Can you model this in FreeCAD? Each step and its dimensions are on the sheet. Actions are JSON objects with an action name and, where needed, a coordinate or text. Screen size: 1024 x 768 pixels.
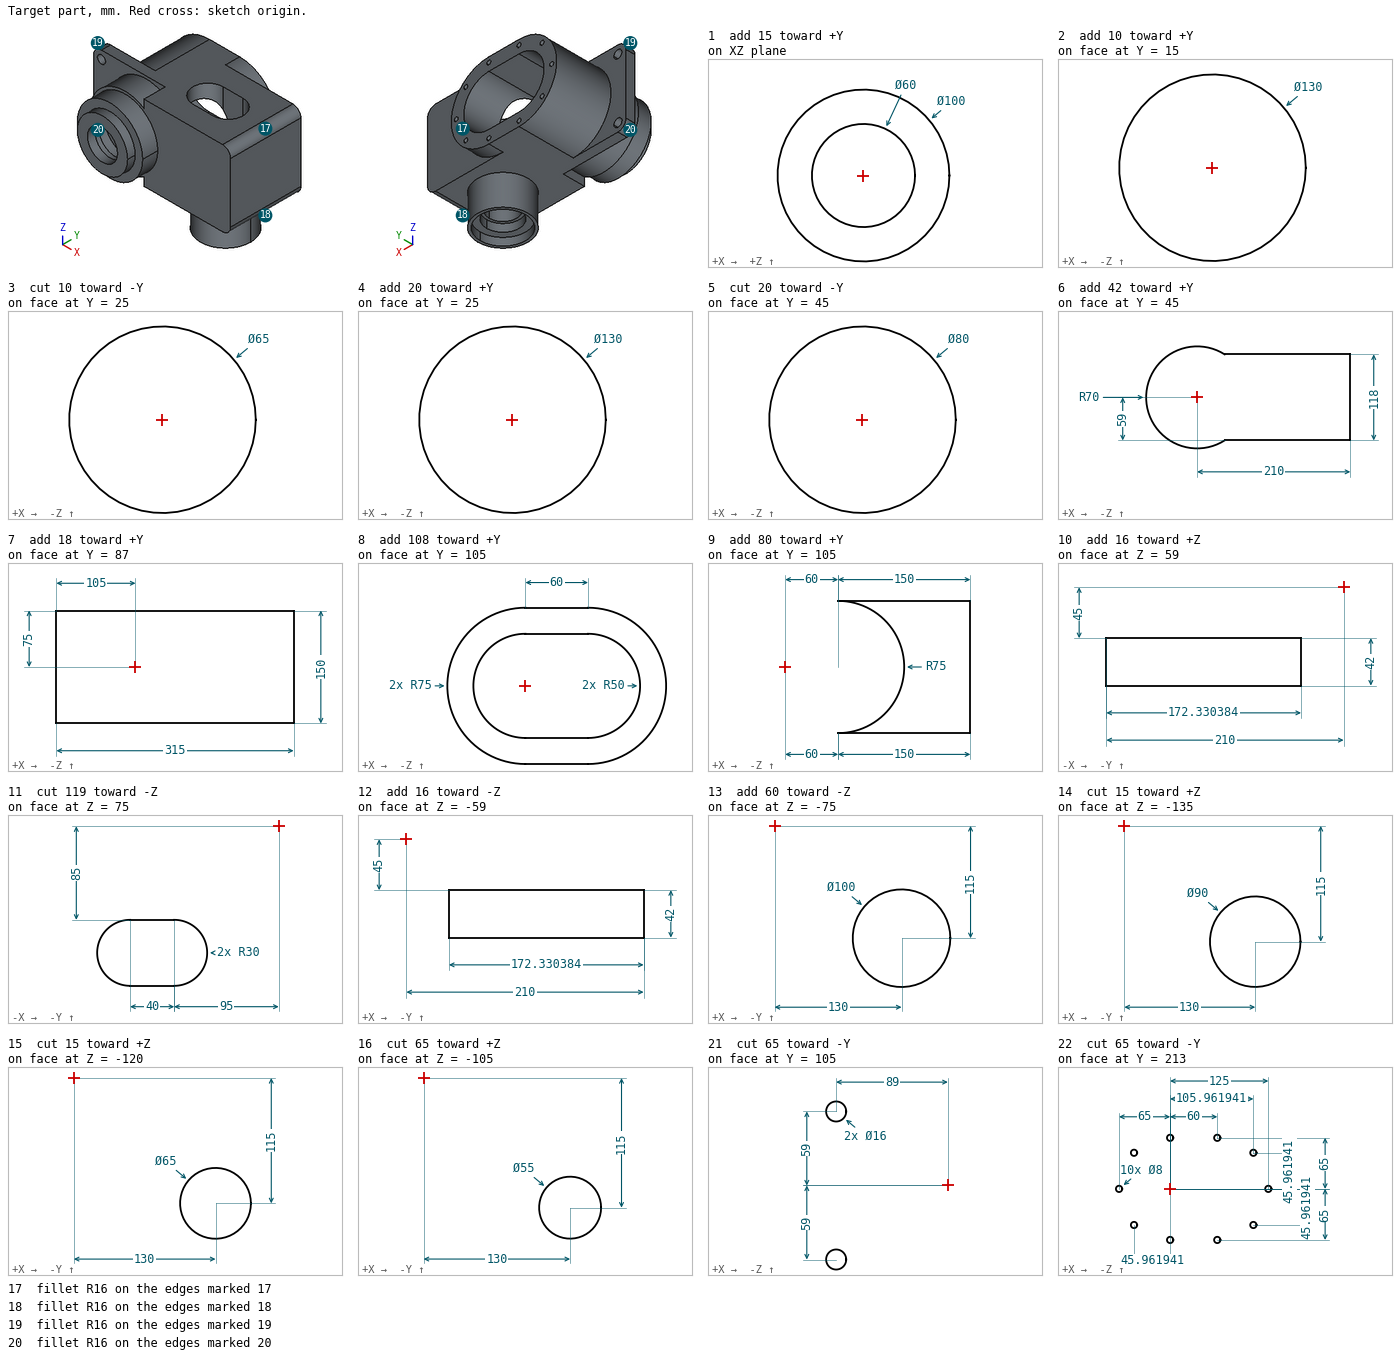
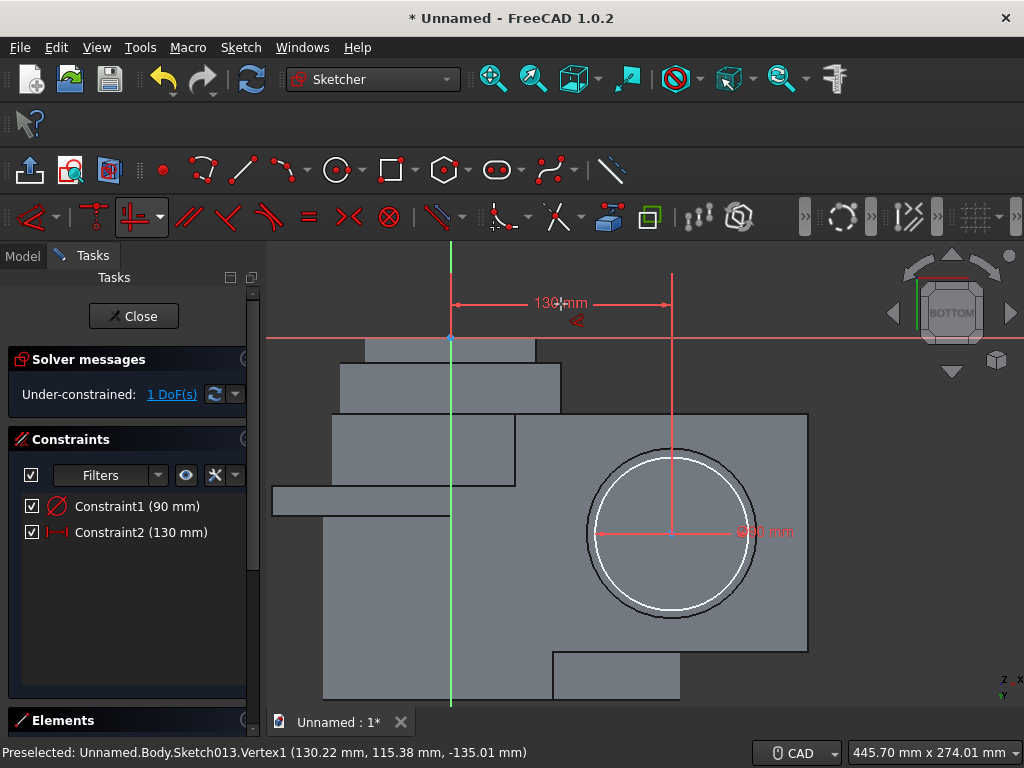
{"action": "left_click", "coordinate": [672, 534]}
{"action": "left_click", "coordinate": [417, 436]}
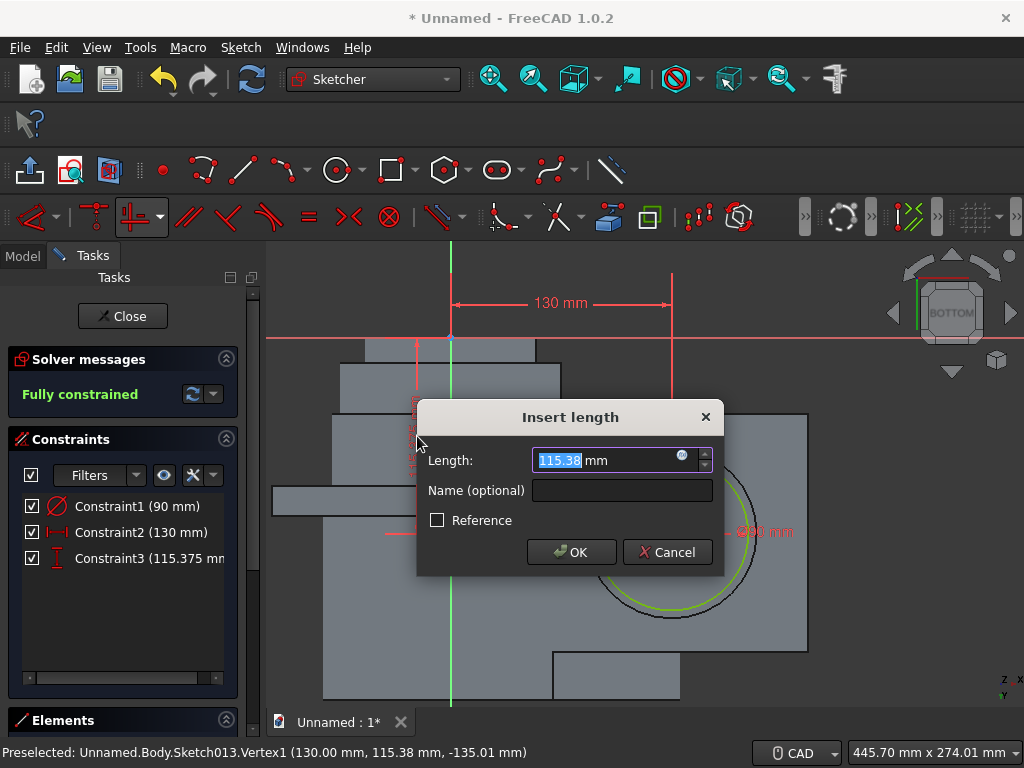
{"action": "type", "text": "115"}
{"action": "key", "text": "Return"}
{"action": "key", "text": "Escape"}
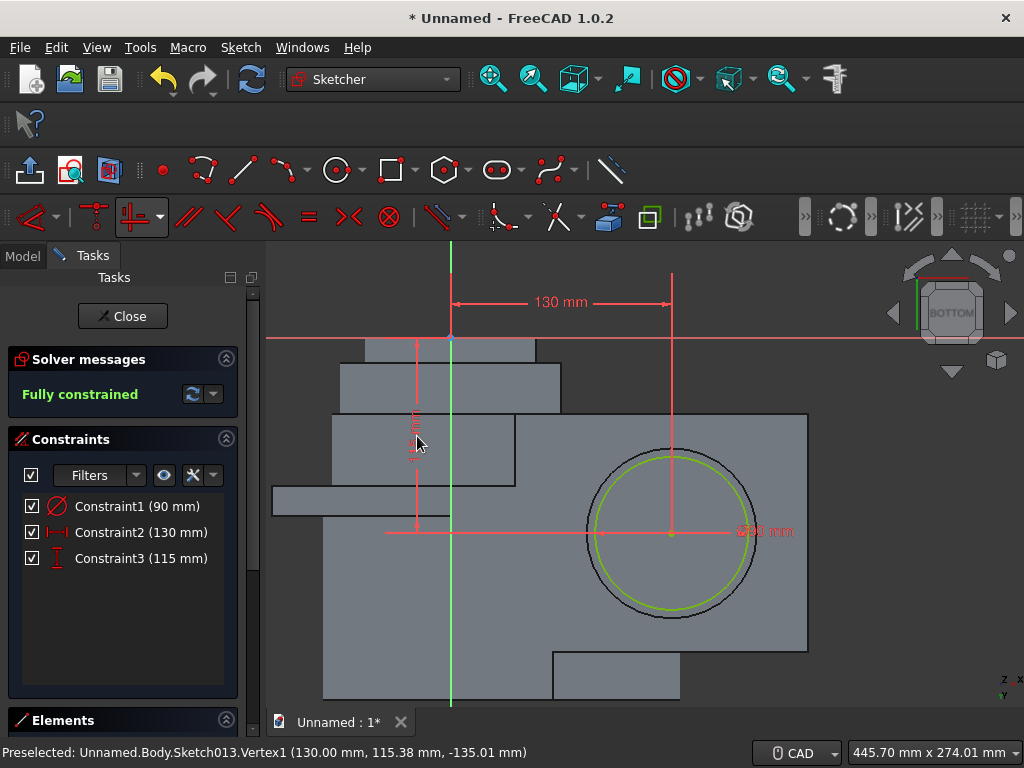
{"action": "left_click", "coordinate": [123, 316]}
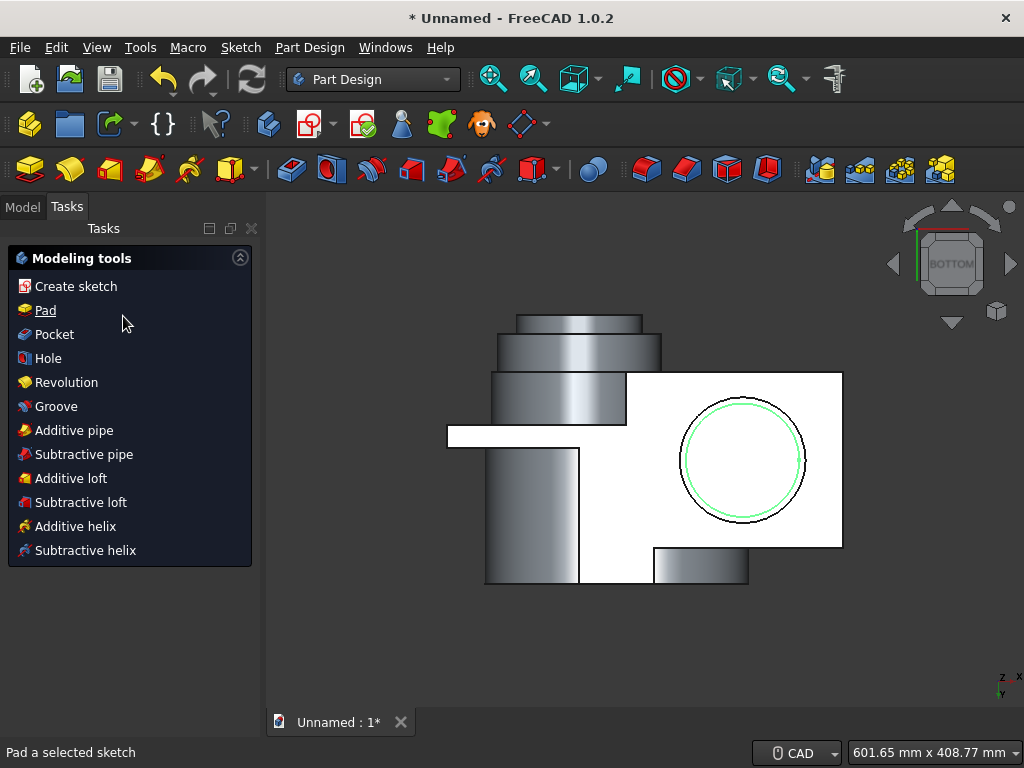
{"action": "left_click", "coordinate": [292, 170]}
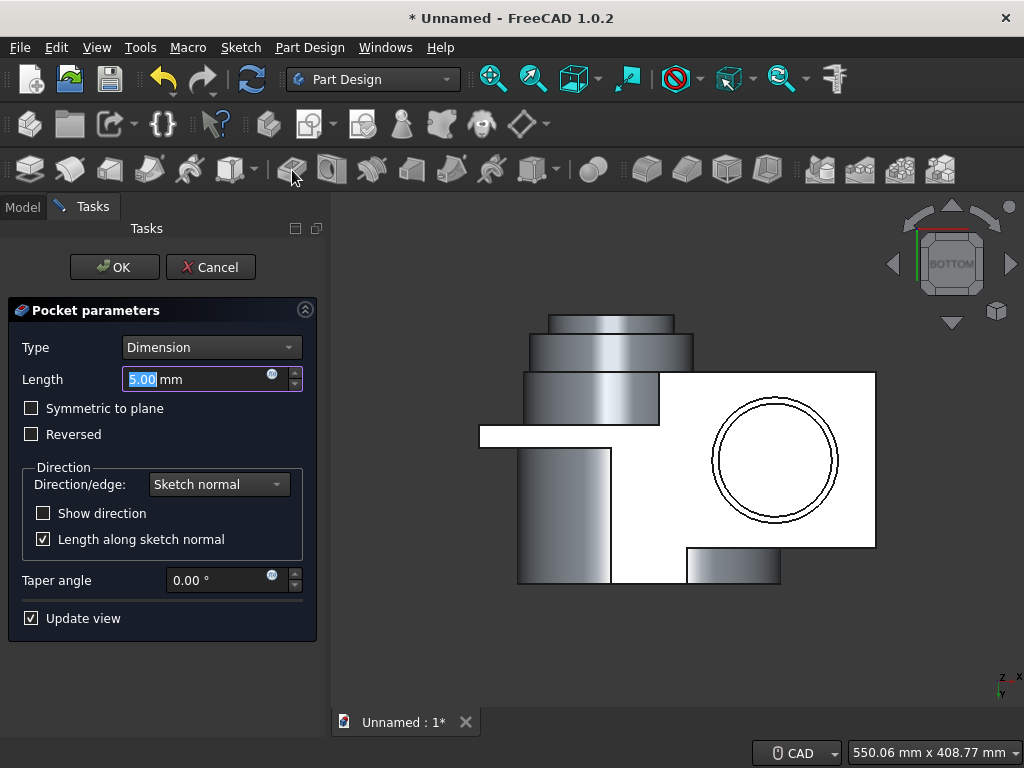
{"action": "type", "text": "15"}
{"action": "key", "text": "Tab"}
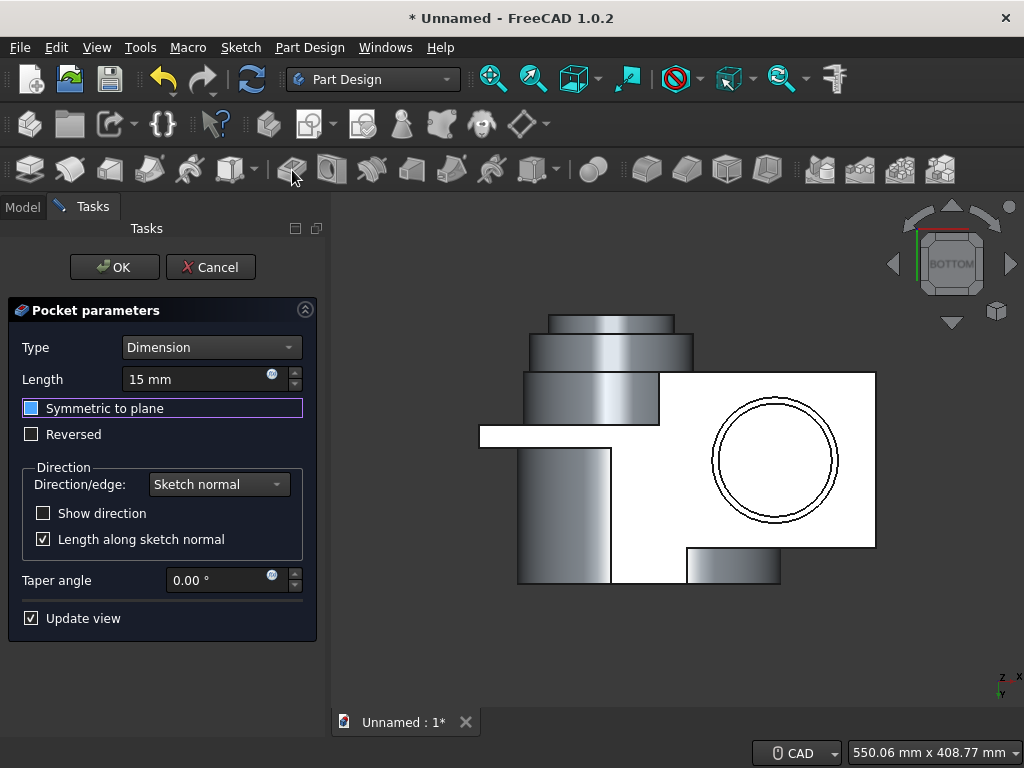
{"action": "left_click", "coordinate": [115, 267]}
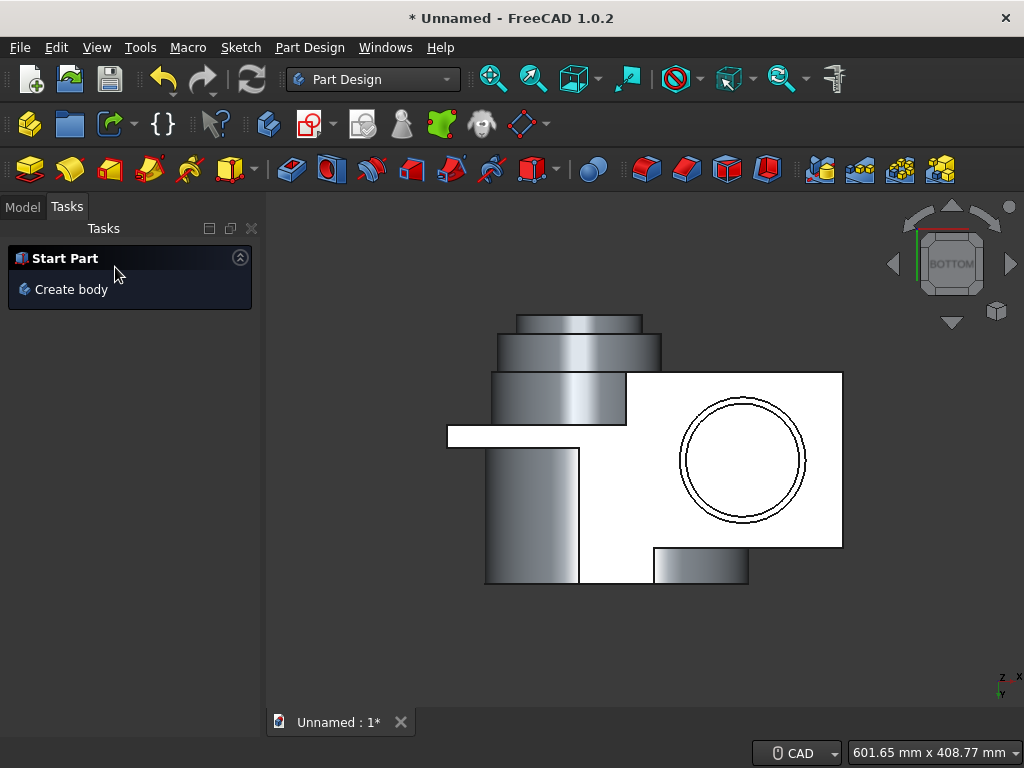
{"action": "left_click", "coordinate": [743, 459]}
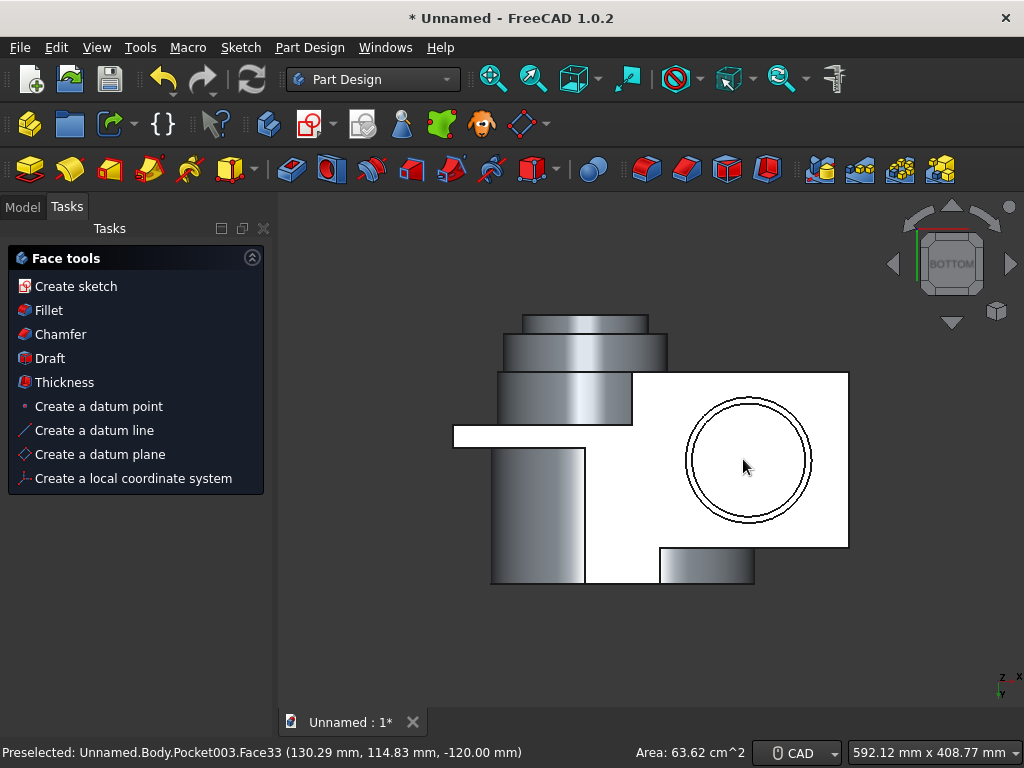
{"action": "left_click", "coordinate": [310, 124]}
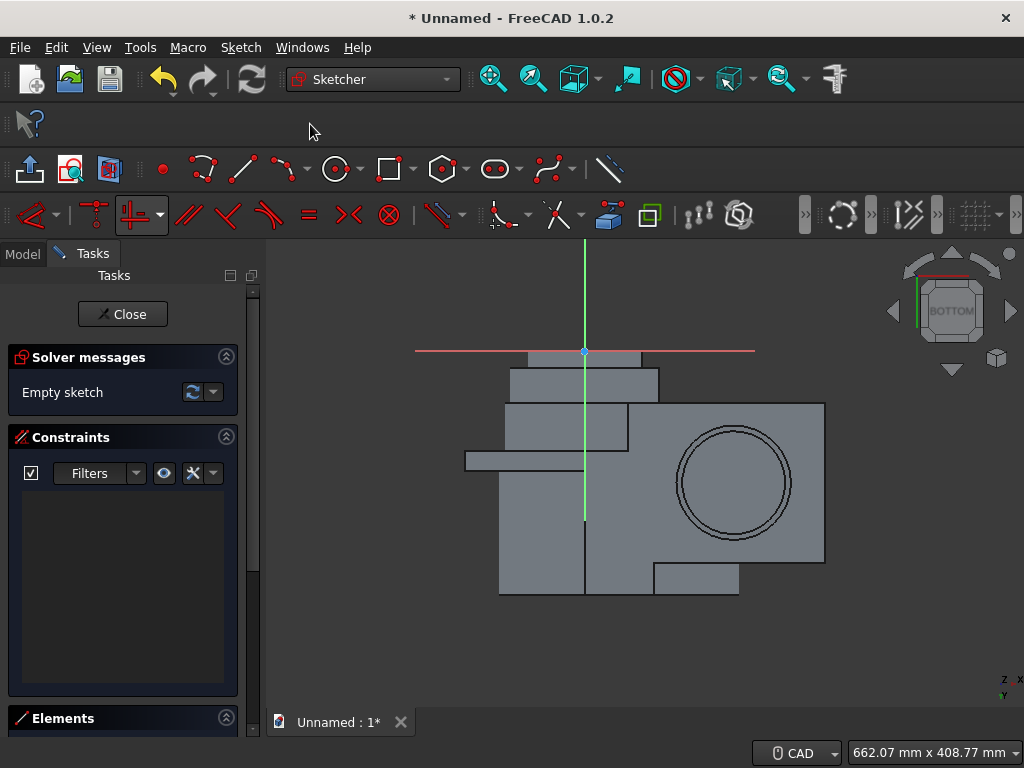
{"action": "left_click", "coordinate": [110, 170]}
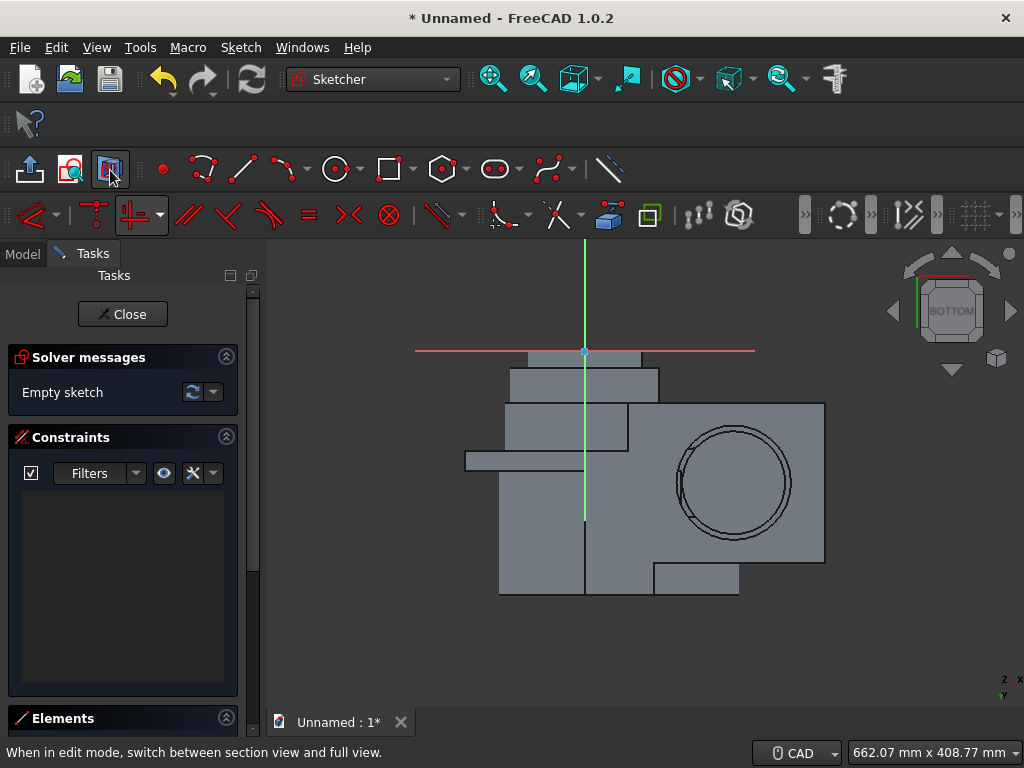
{"action": "scroll", "coordinate": [785, 486], "scroll_direction": "up", "scroll_amount": 7}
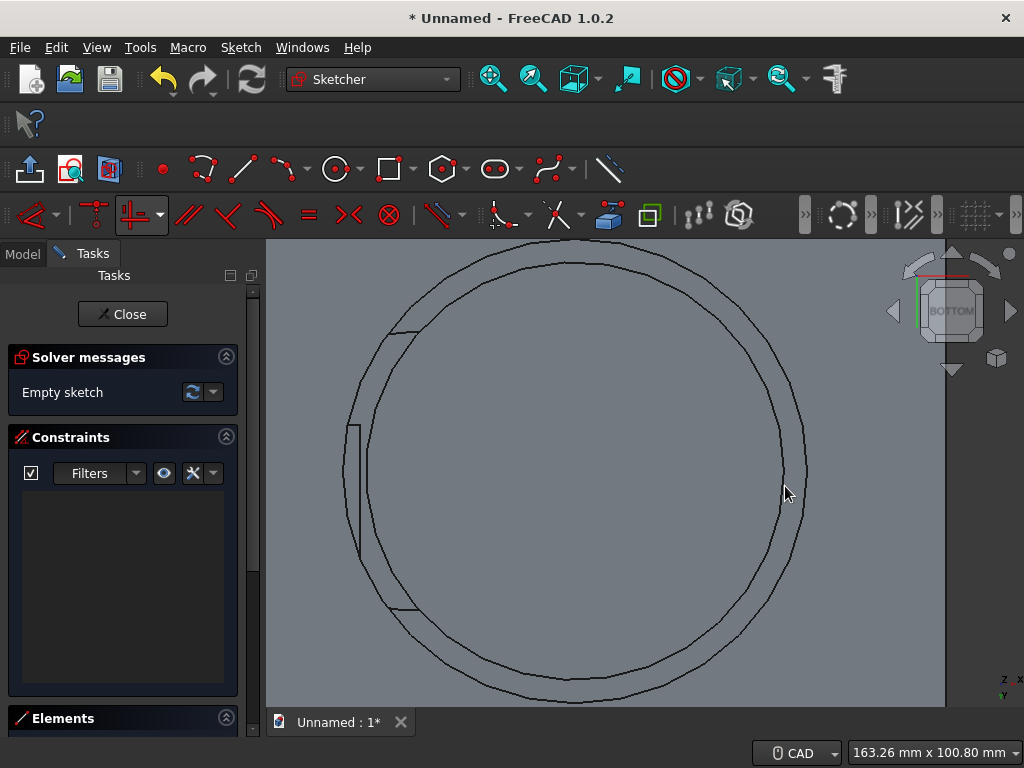
{"action": "left_click", "coordinate": [336, 170]}